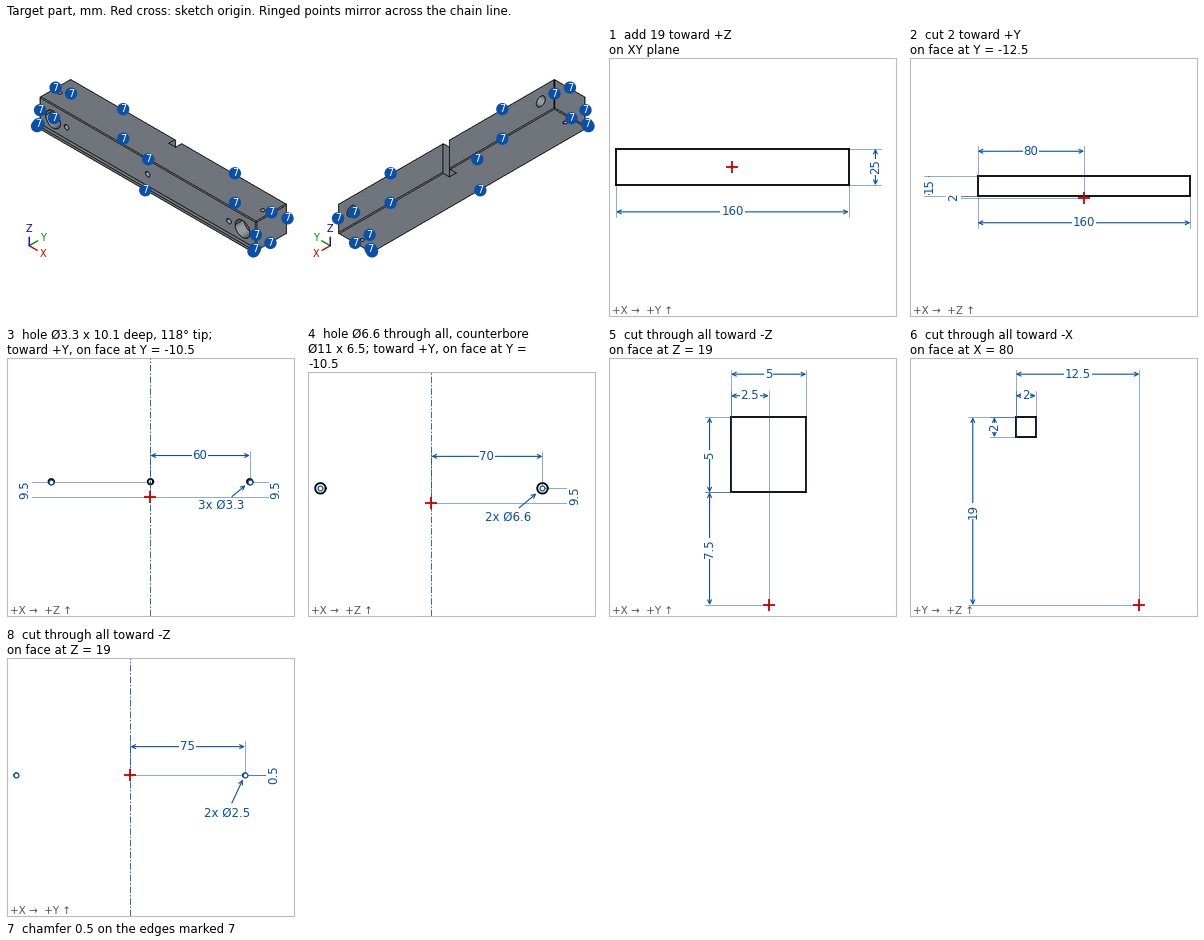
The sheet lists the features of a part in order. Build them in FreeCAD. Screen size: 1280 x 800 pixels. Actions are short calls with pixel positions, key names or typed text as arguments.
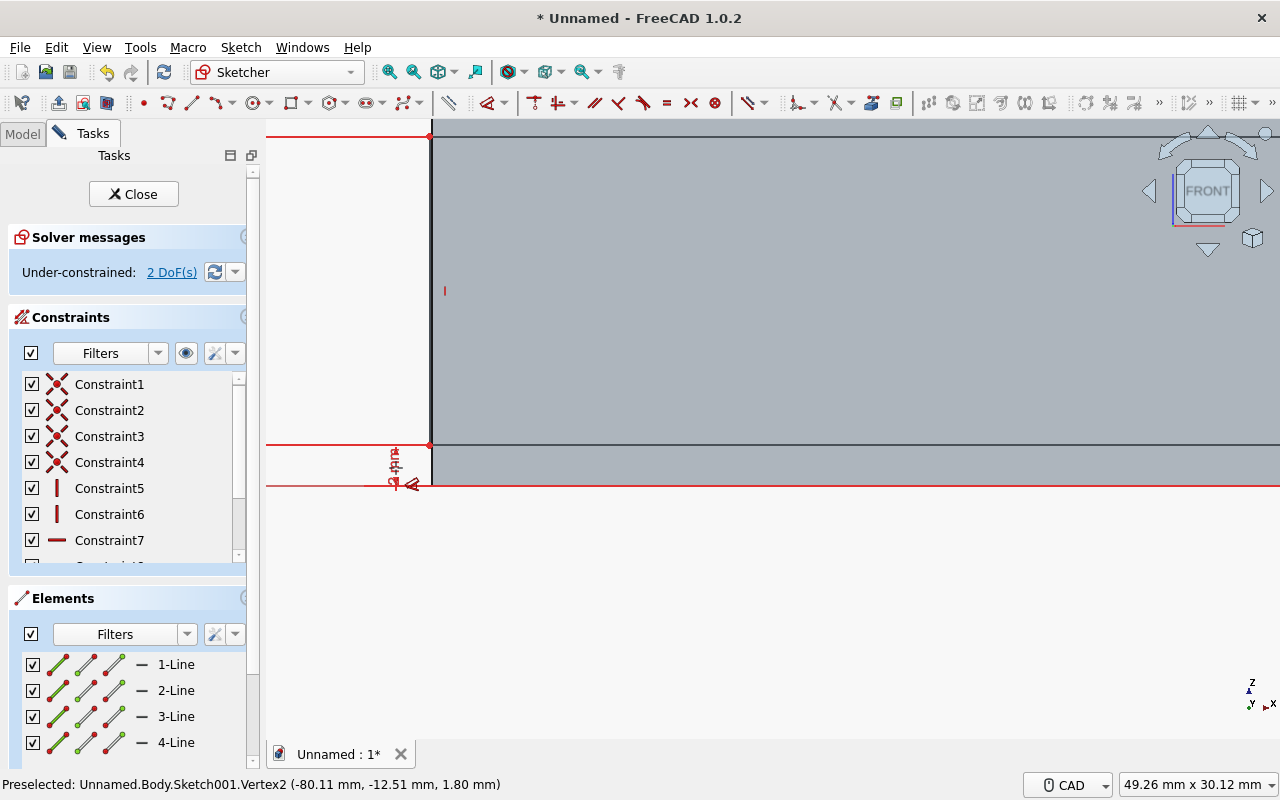
scroll(432, 452, down, 9)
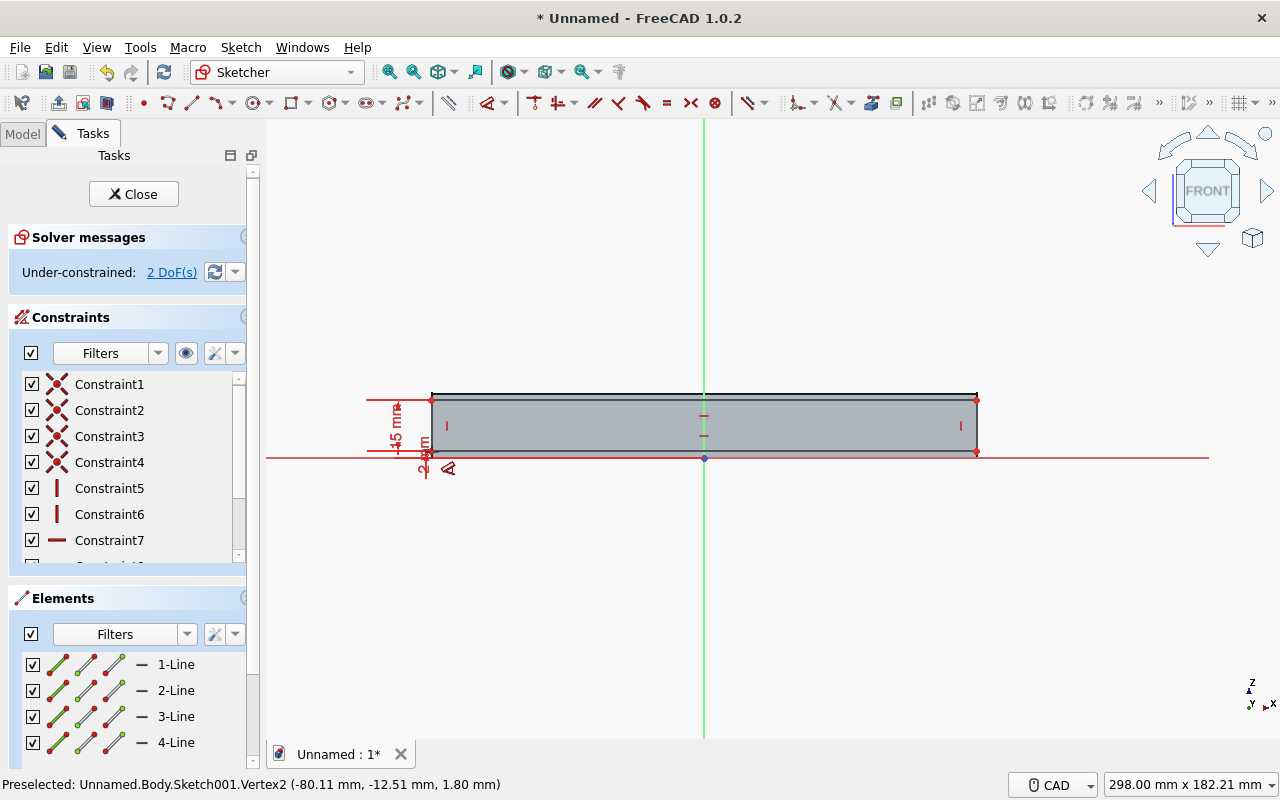
scroll(541, 451, up, 4)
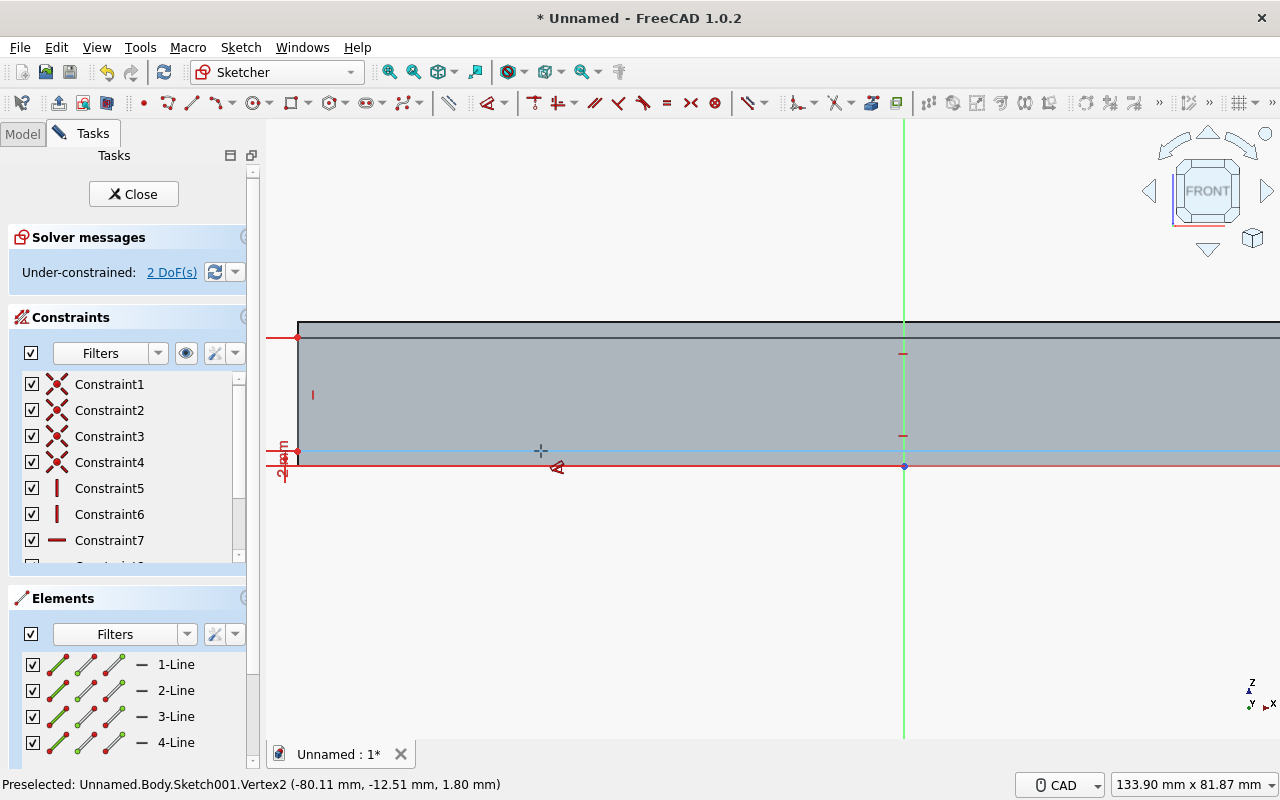
click(540, 451)
click(706, 485)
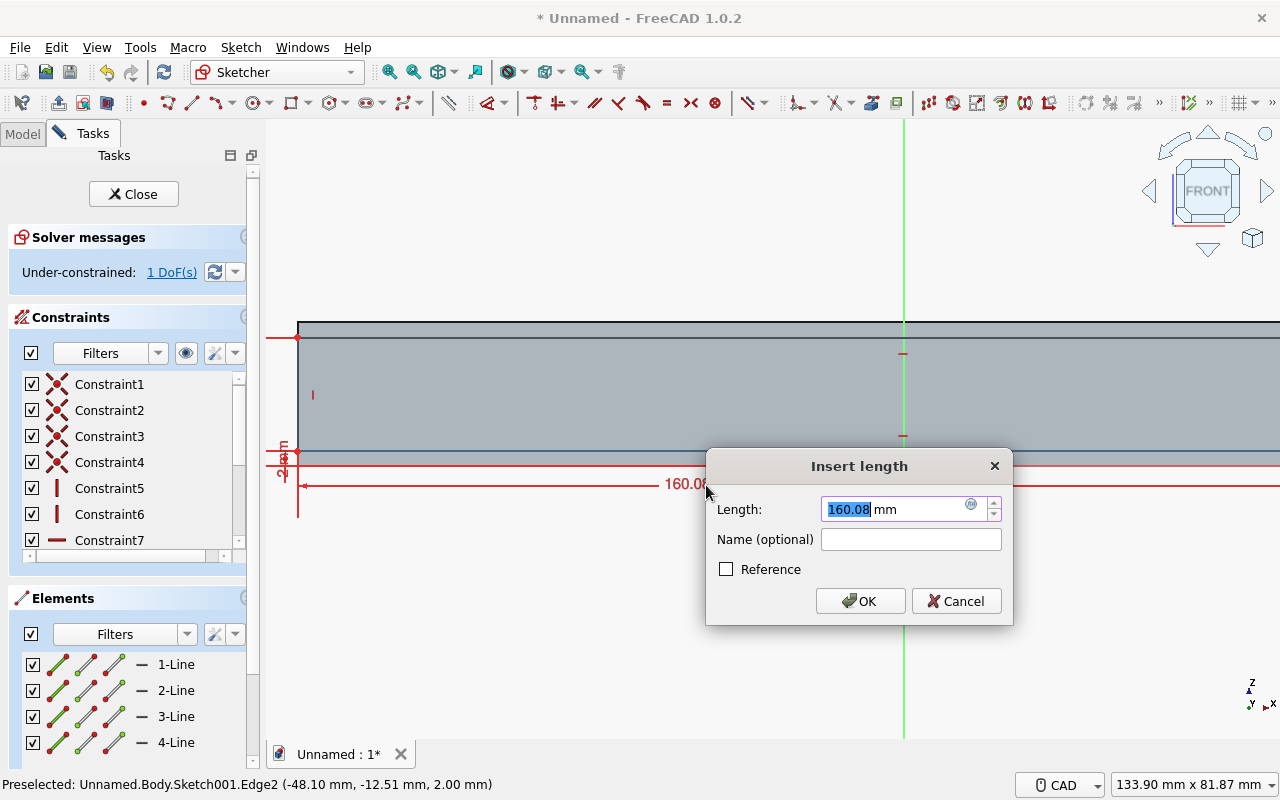
text(160)
key(Return)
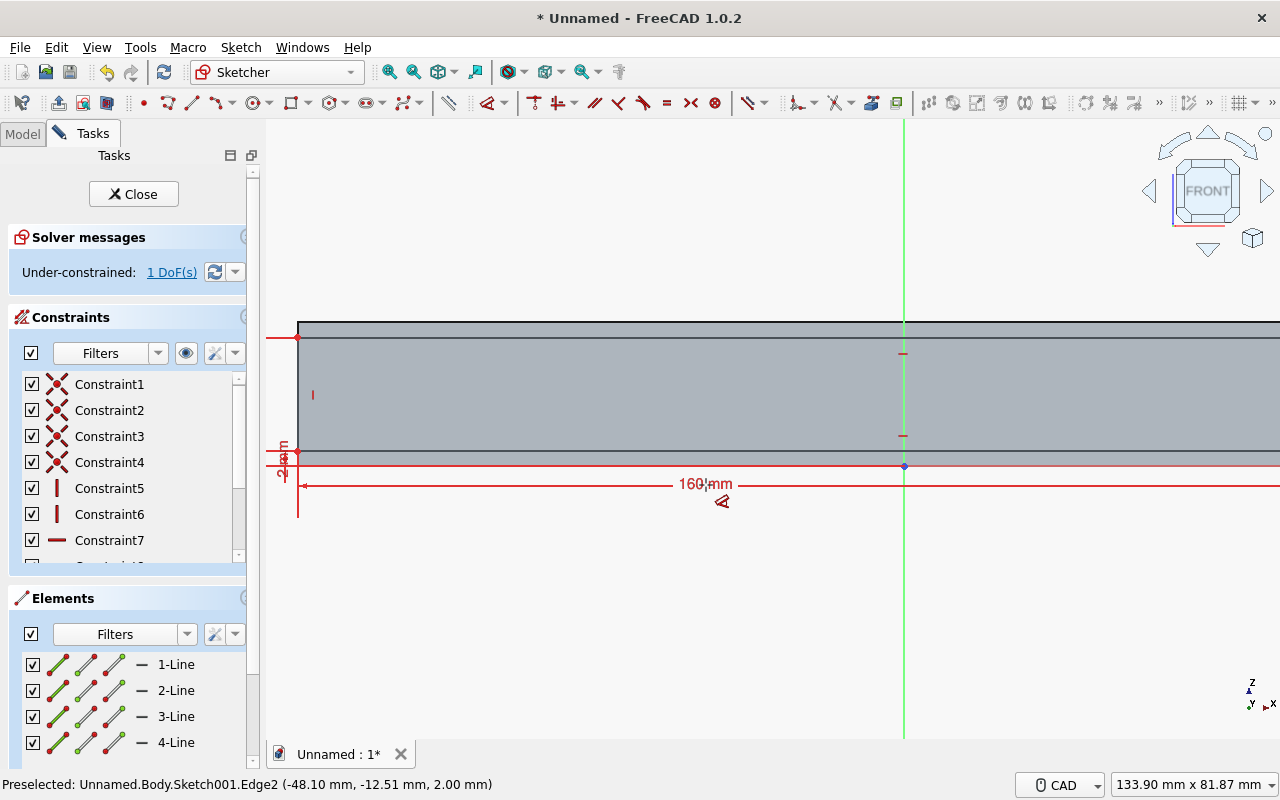
click(298, 338)
click(601, 500)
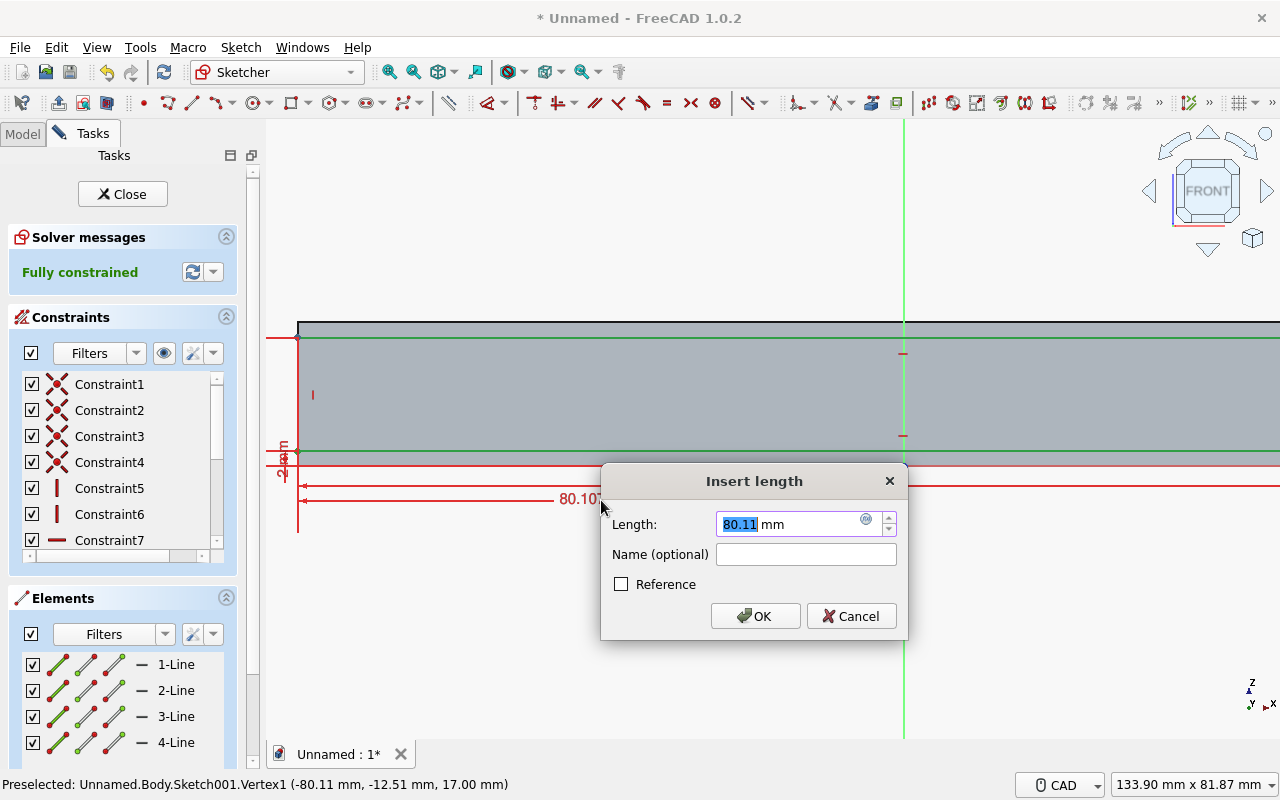
text(80)
key(Return)
key(Escape)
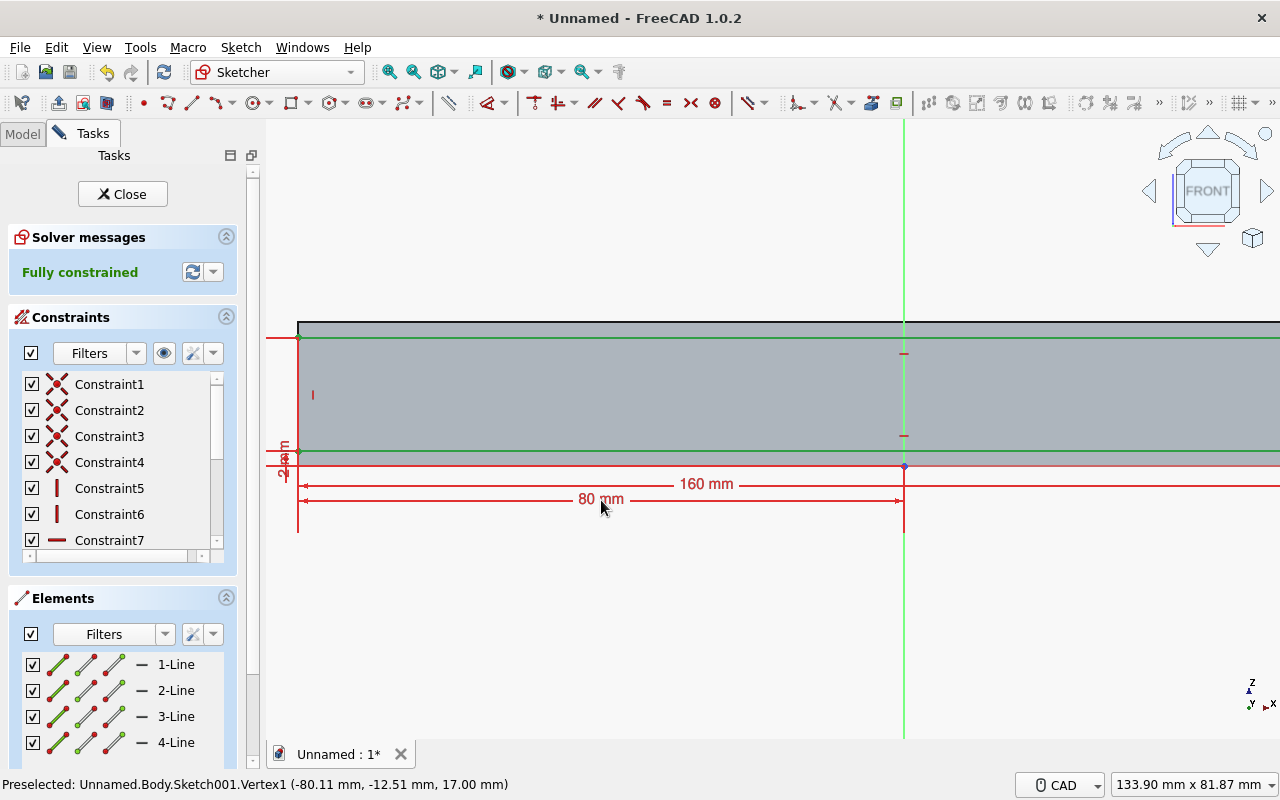
click(123, 194)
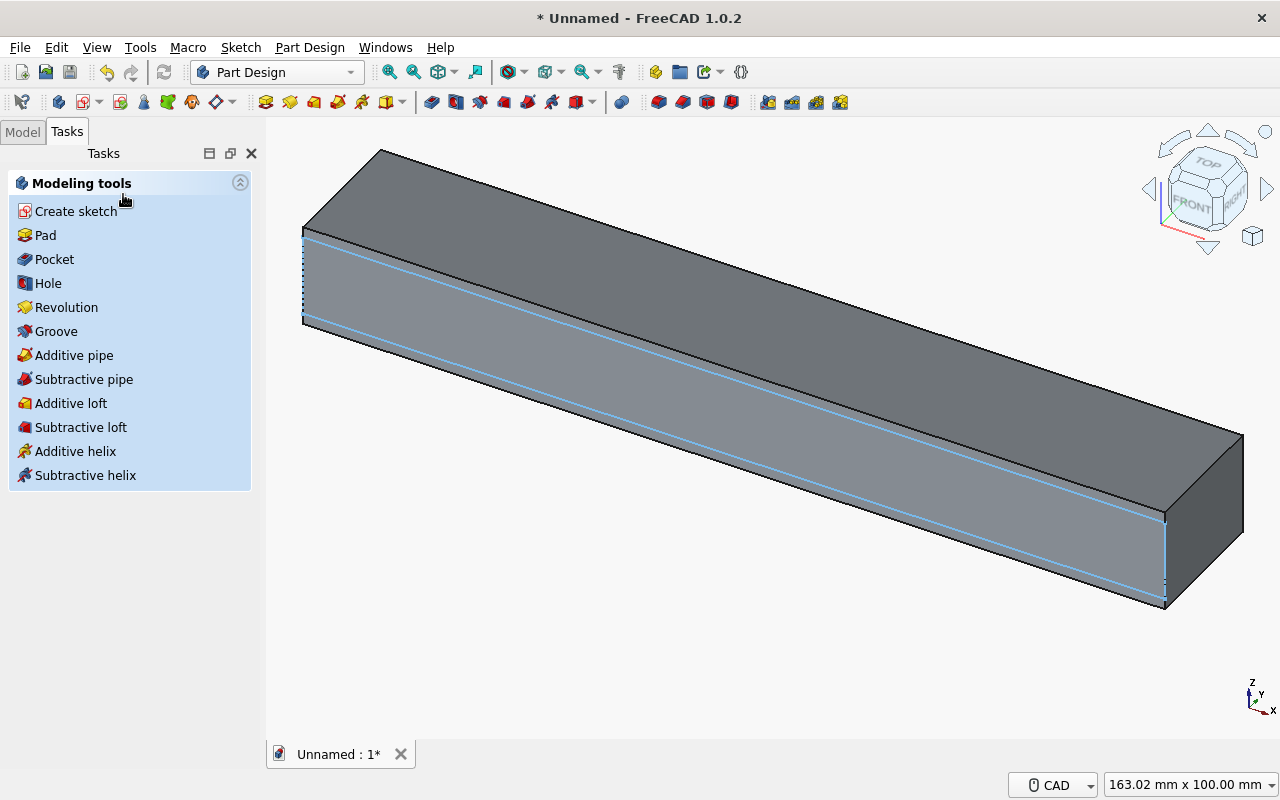
click(432, 102)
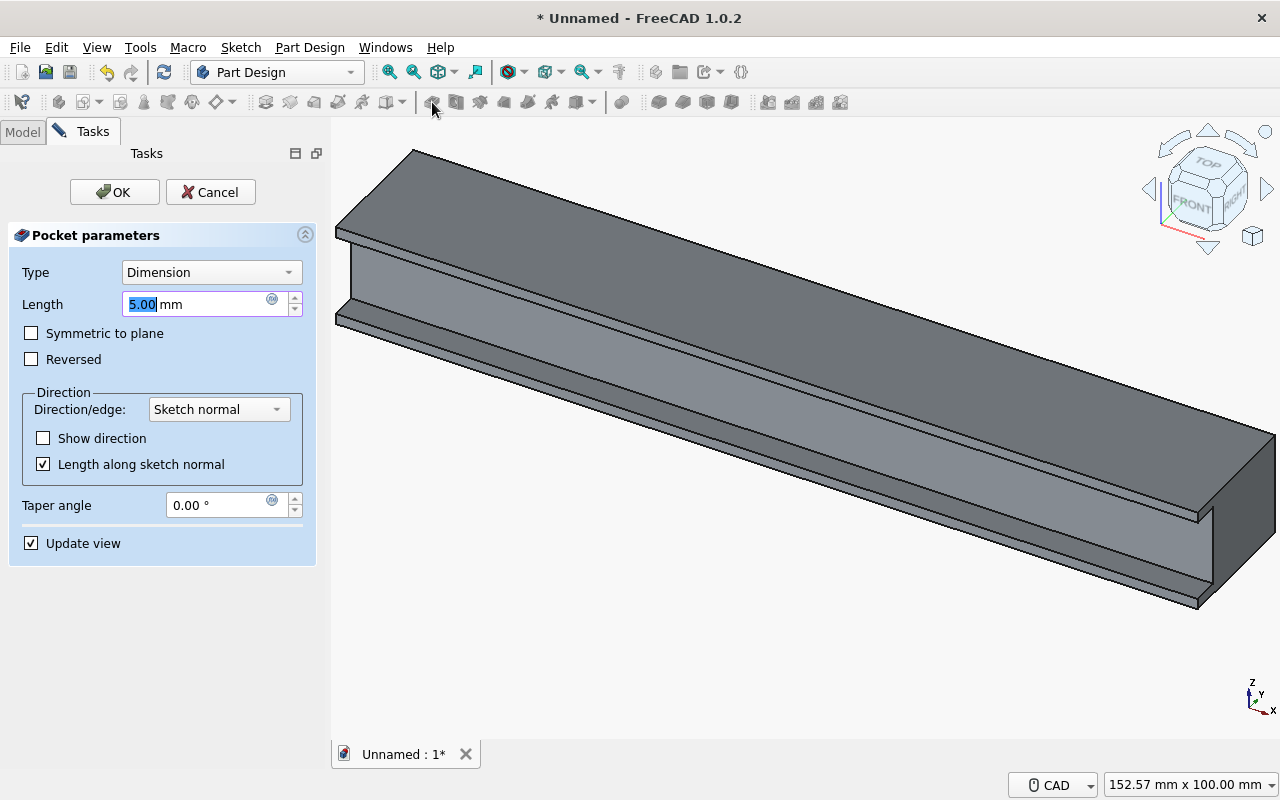
text(2)
key(Tab)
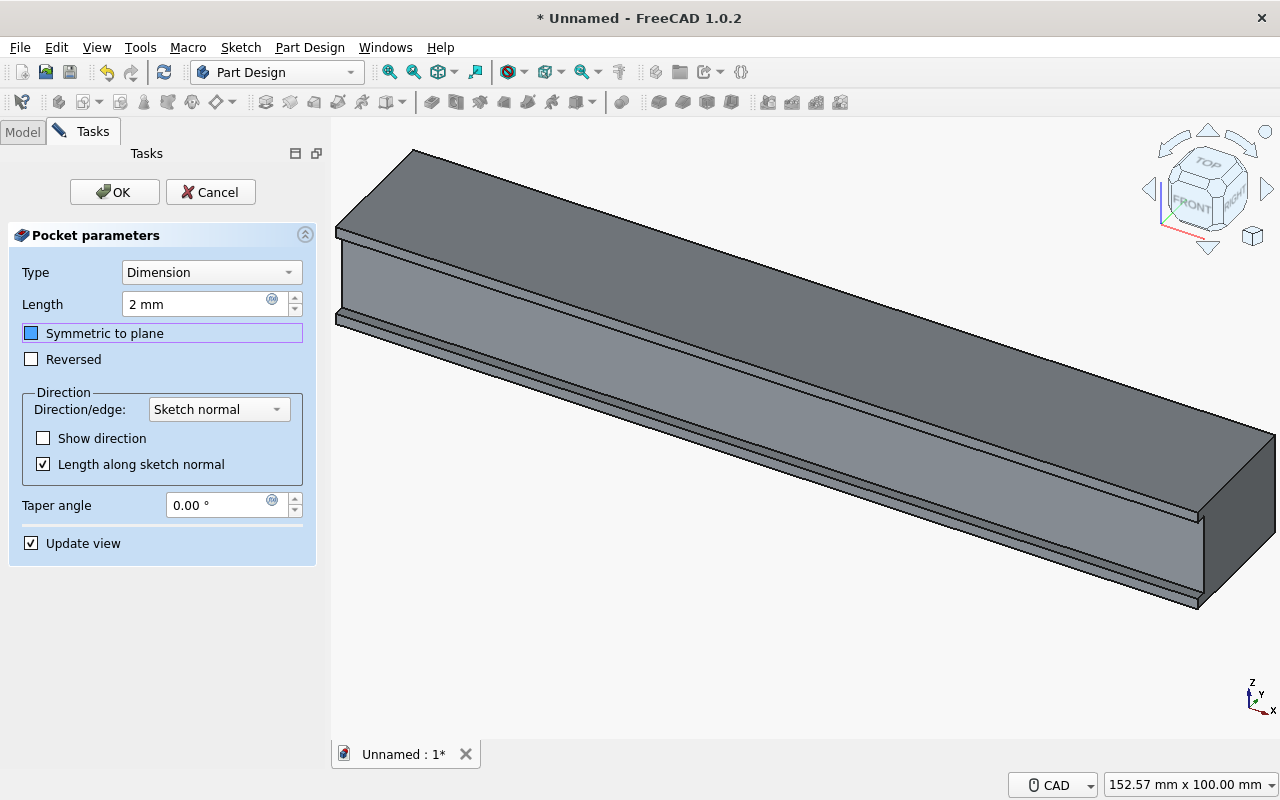
click(115, 192)